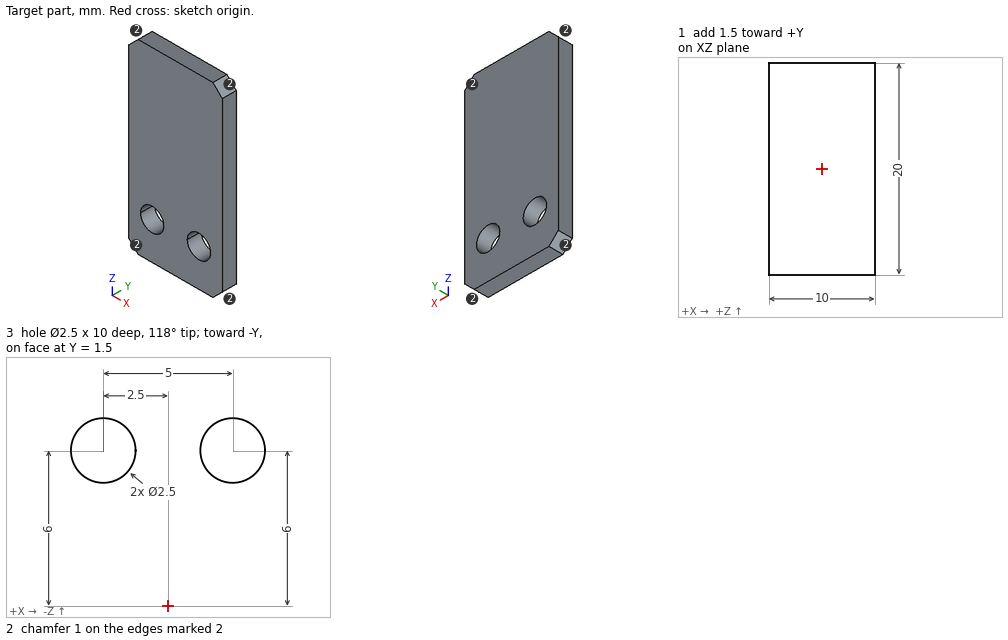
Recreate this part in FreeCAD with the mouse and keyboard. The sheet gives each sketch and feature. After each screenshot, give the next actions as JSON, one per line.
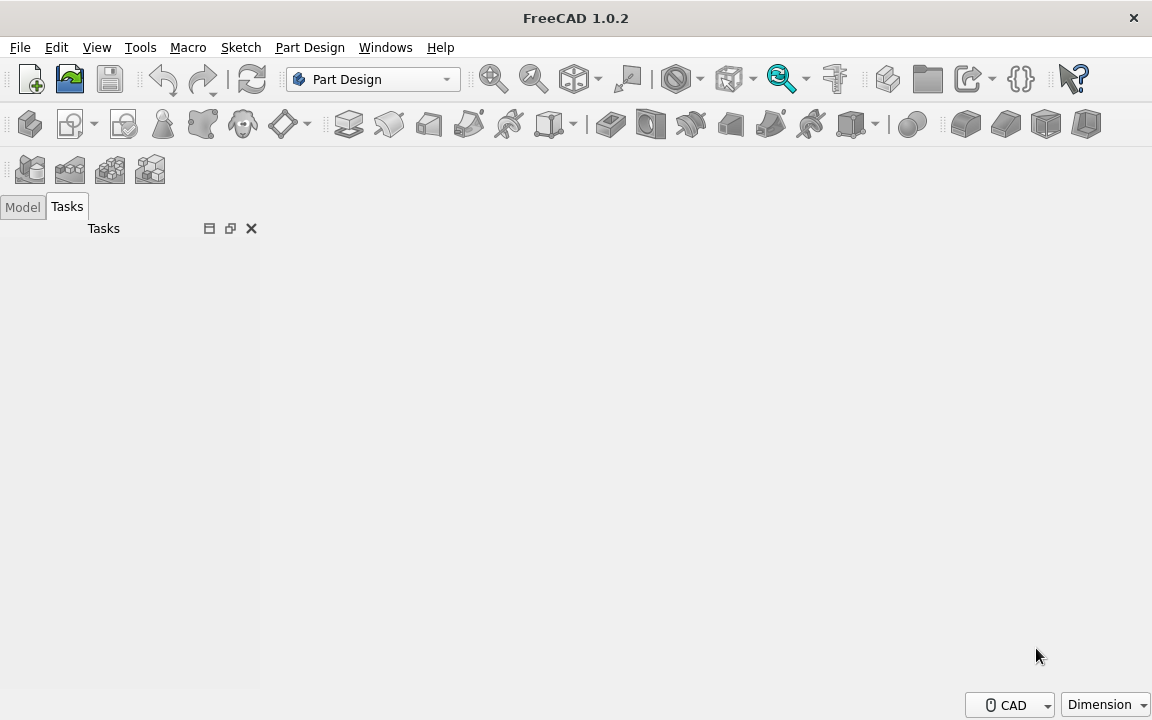
{"action": "left_click", "coordinate": [30, 80]}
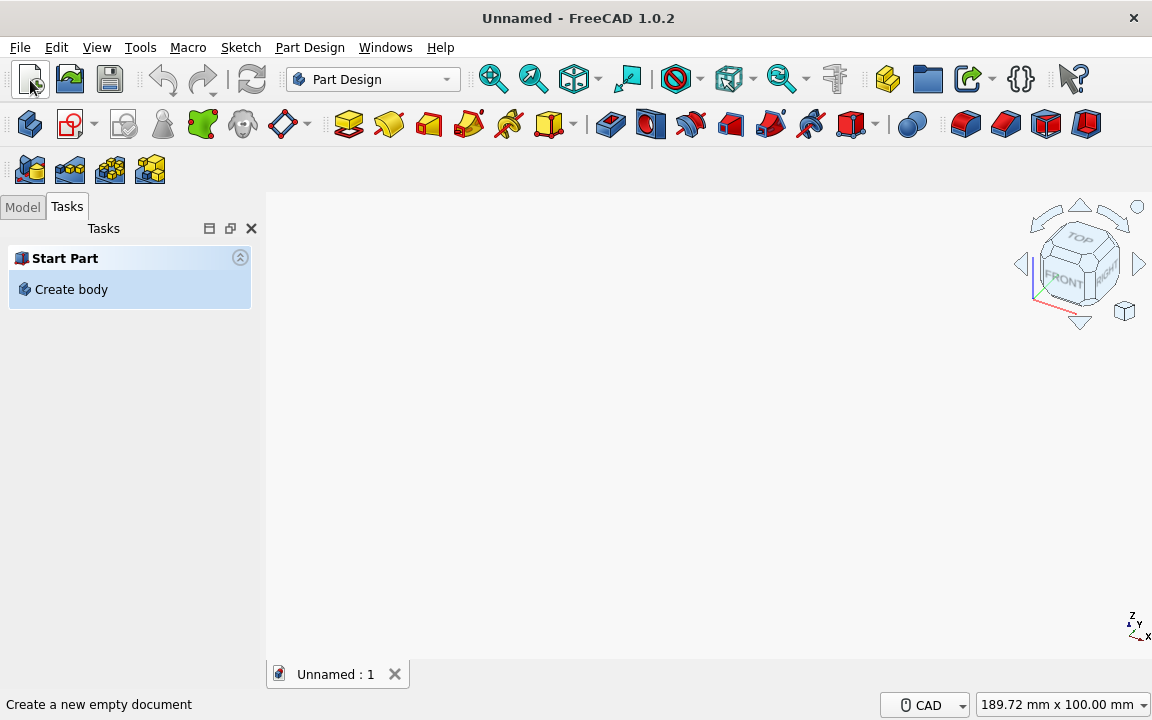
{"action": "left_click", "coordinate": [70, 124]}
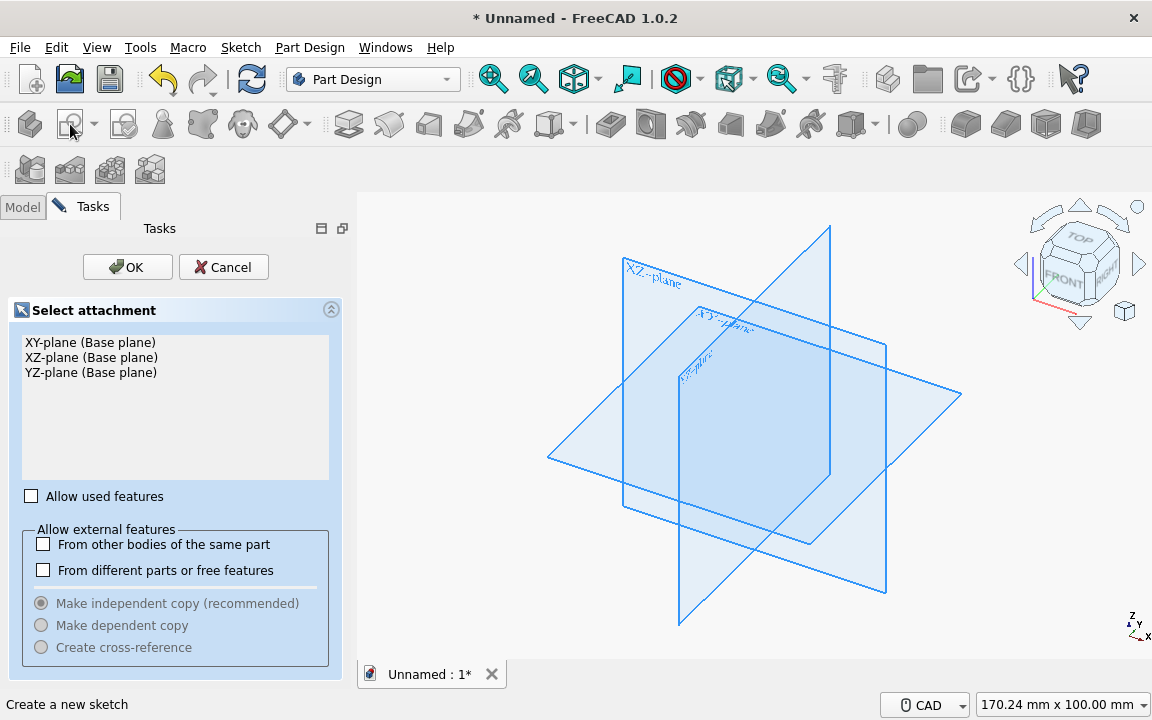
{"action": "left_click", "coordinate": [82, 358]}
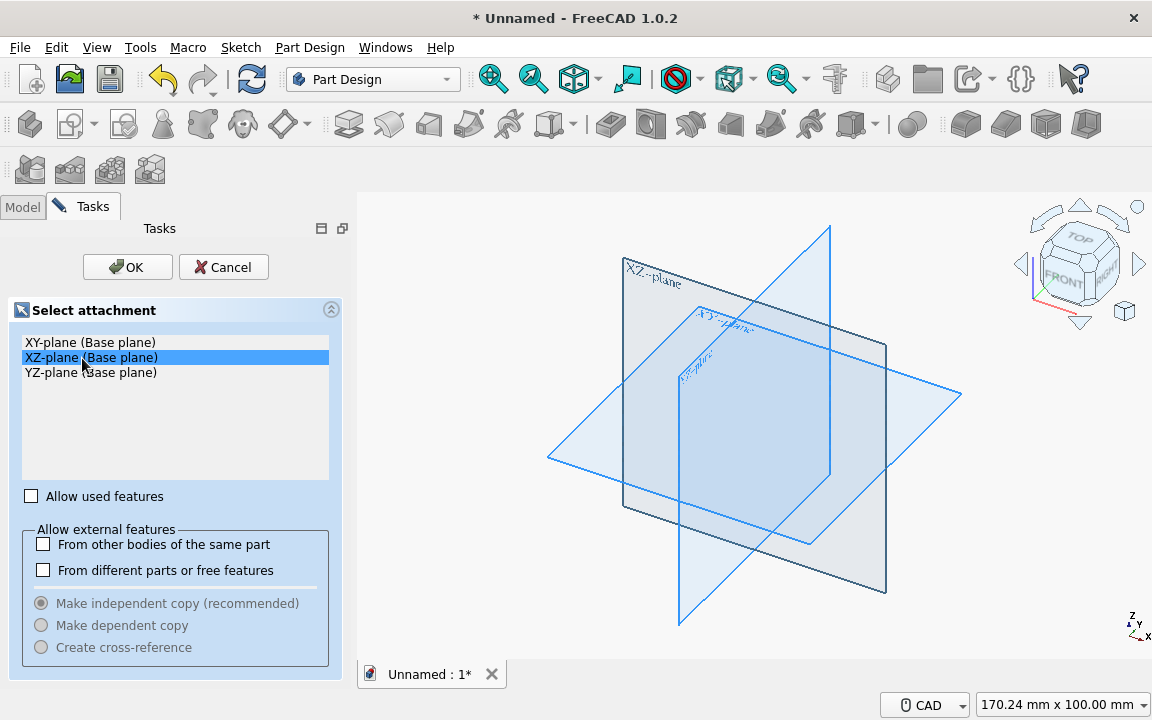
{"action": "left_click", "coordinate": [128, 267]}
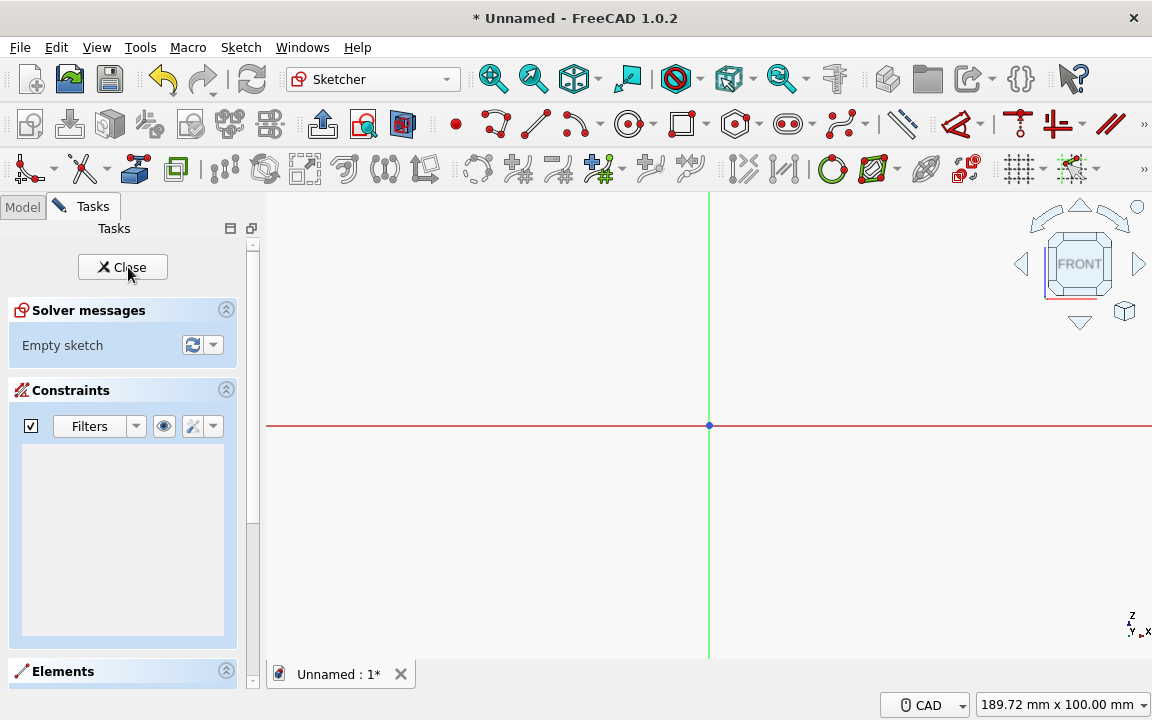
{"action": "scroll", "coordinate": [739, 426], "scroll_direction": "up", "scroll_amount": 6}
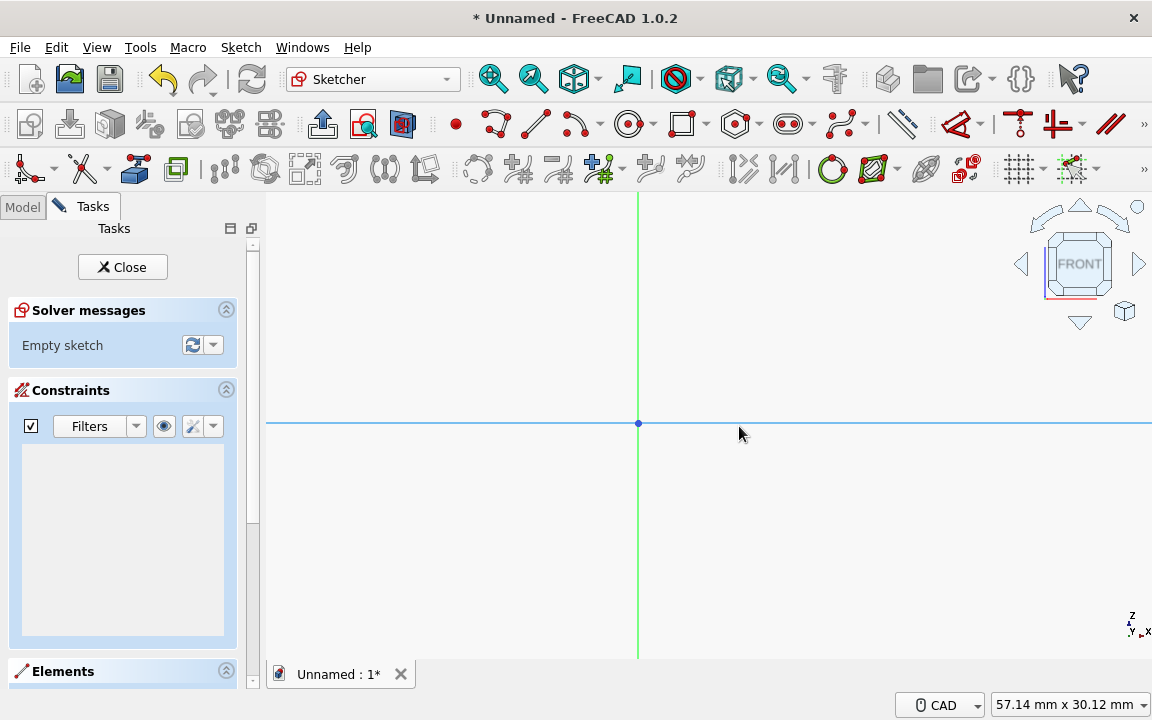
{"action": "left_click", "coordinate": [708, 124]}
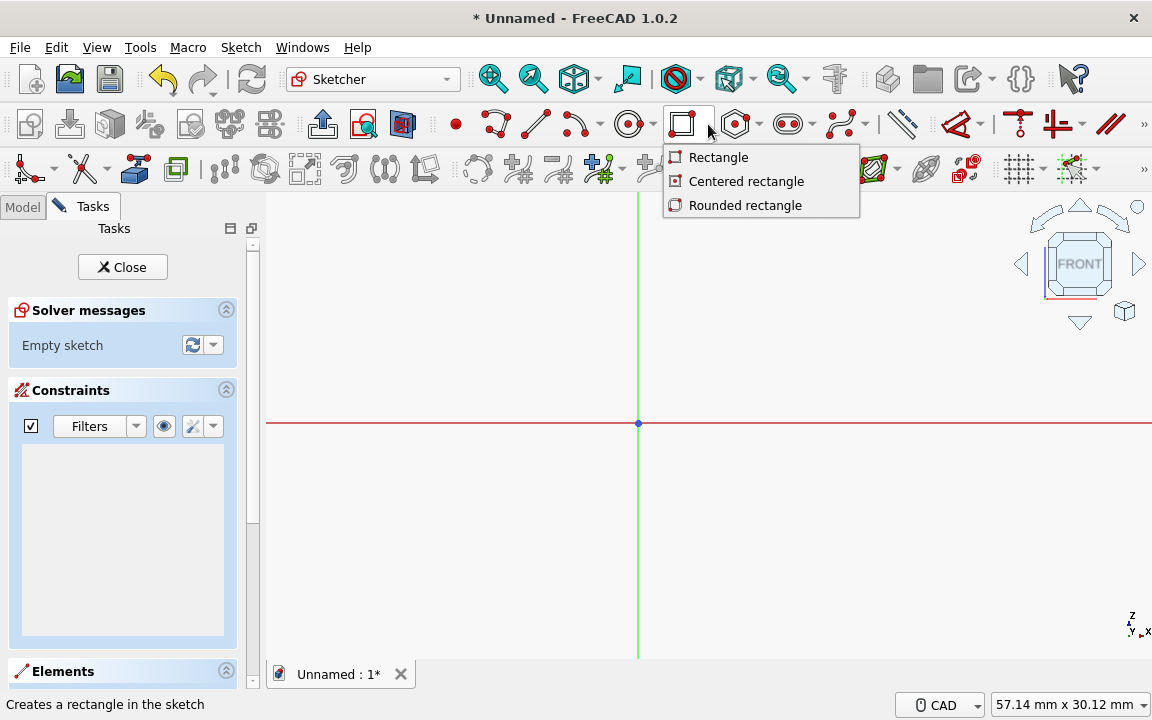
{"action": "left_click", "coordinate": [762, 181]}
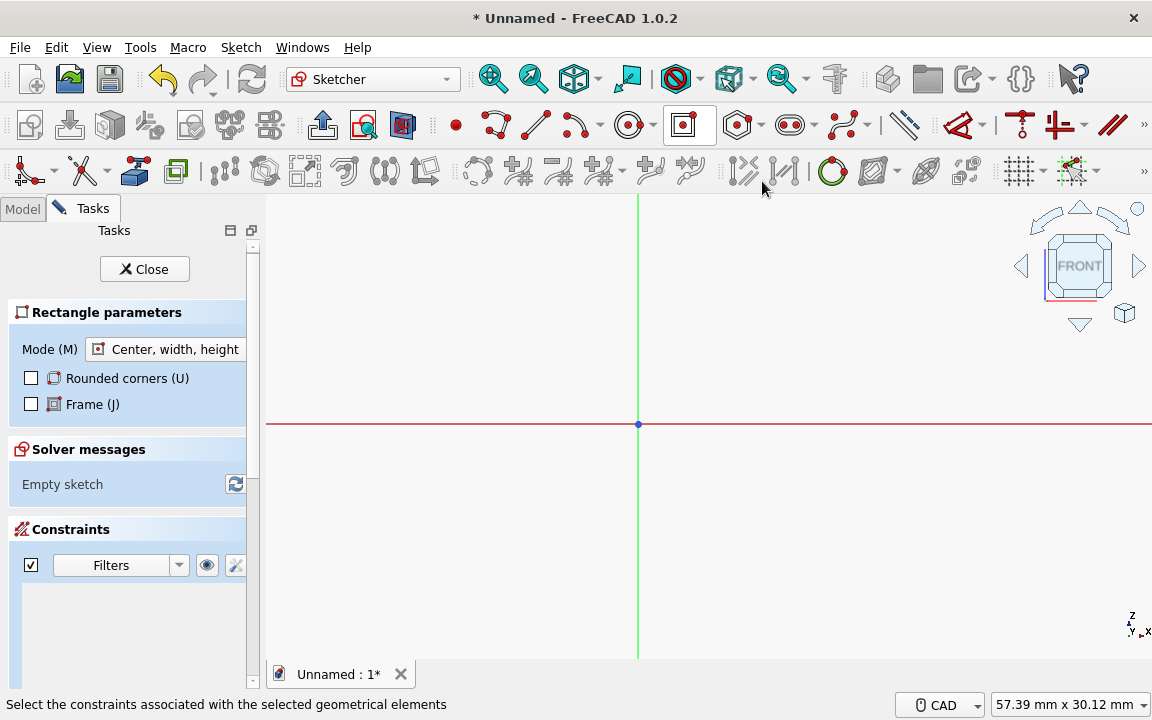
{"action": "left_click", "coordinate": [638, 424]}
{"action": "left_click", "coordinate": [716, 270]}
{"action": "key", "text": "Escape"}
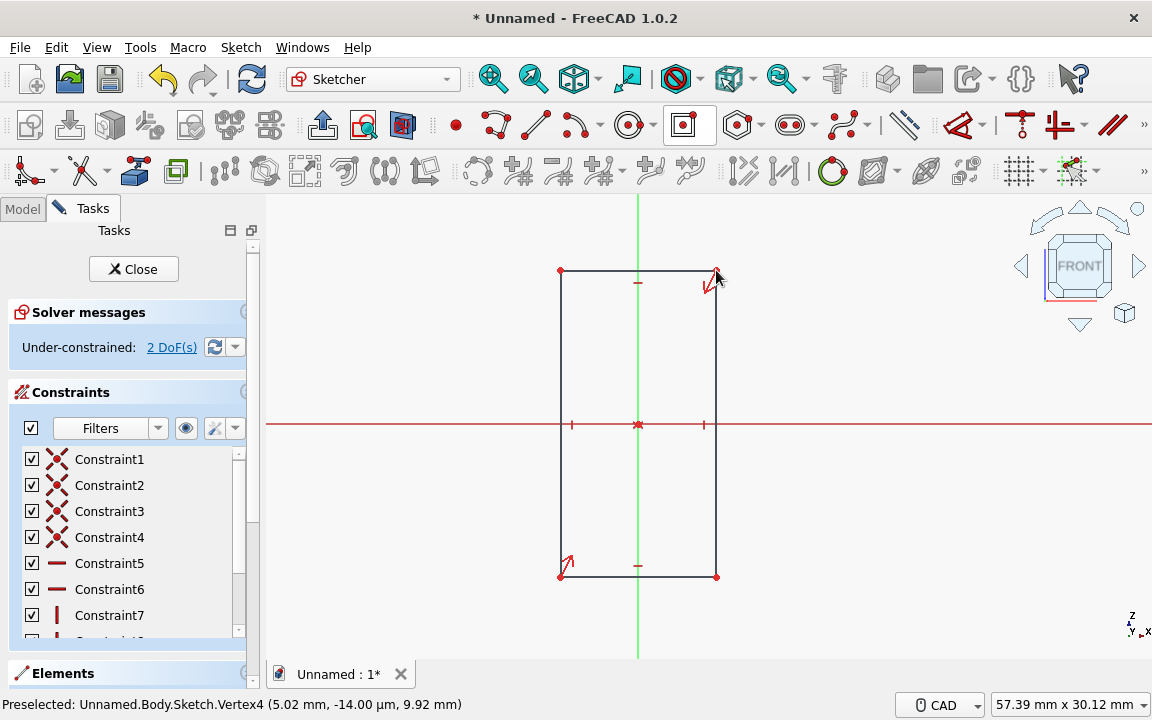
{"action": "left_click", "coordinate": [958, 126]}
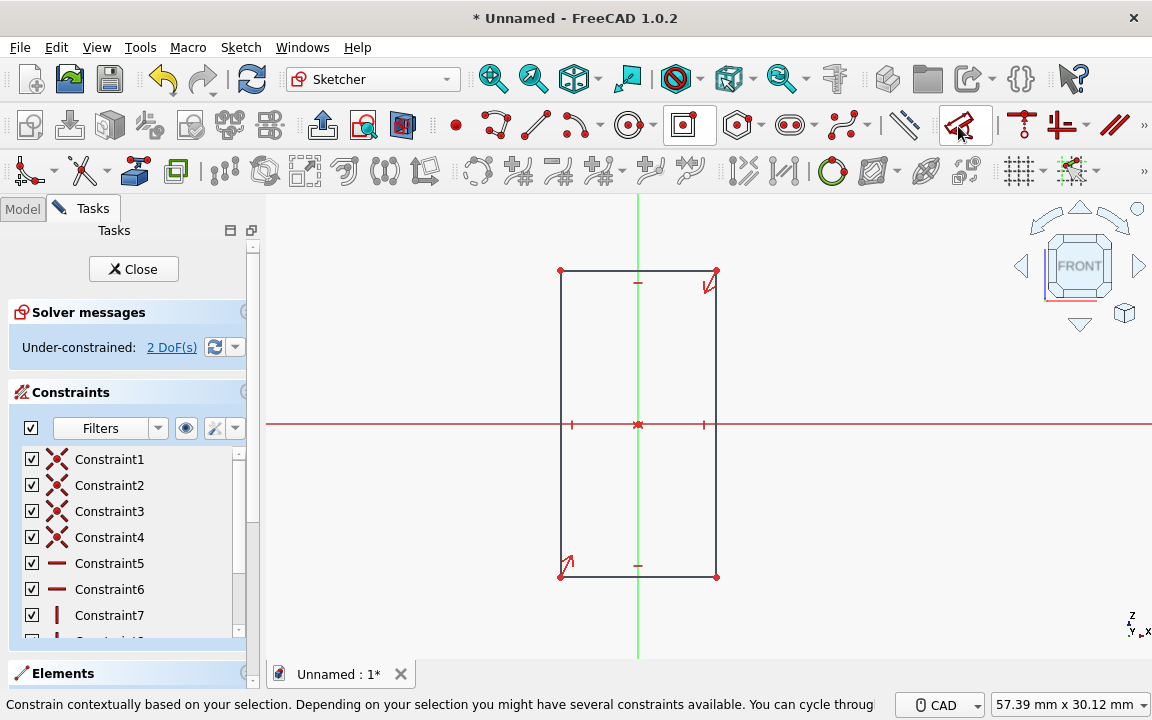
{"action": "left_click", "coordinate": [607, 577]}
{"action": "left_click", "coordinate": [603, 611]}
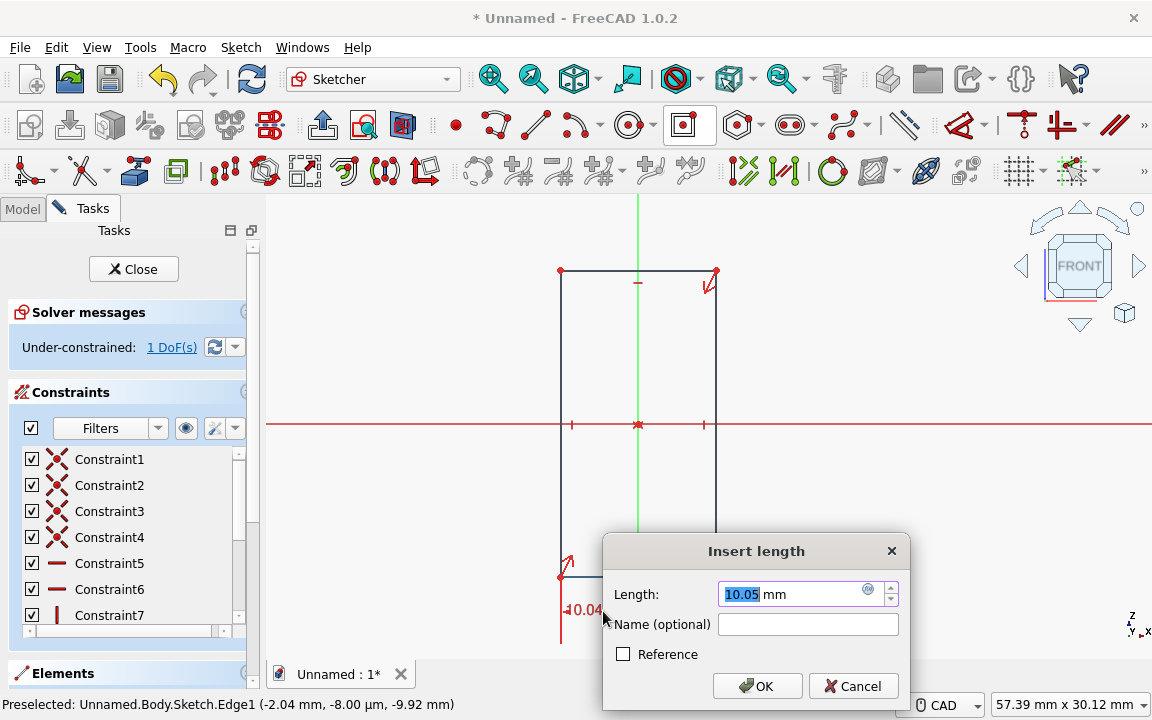
{"action": "type", "text": "10"}
{"action": "key", "text": "Return"}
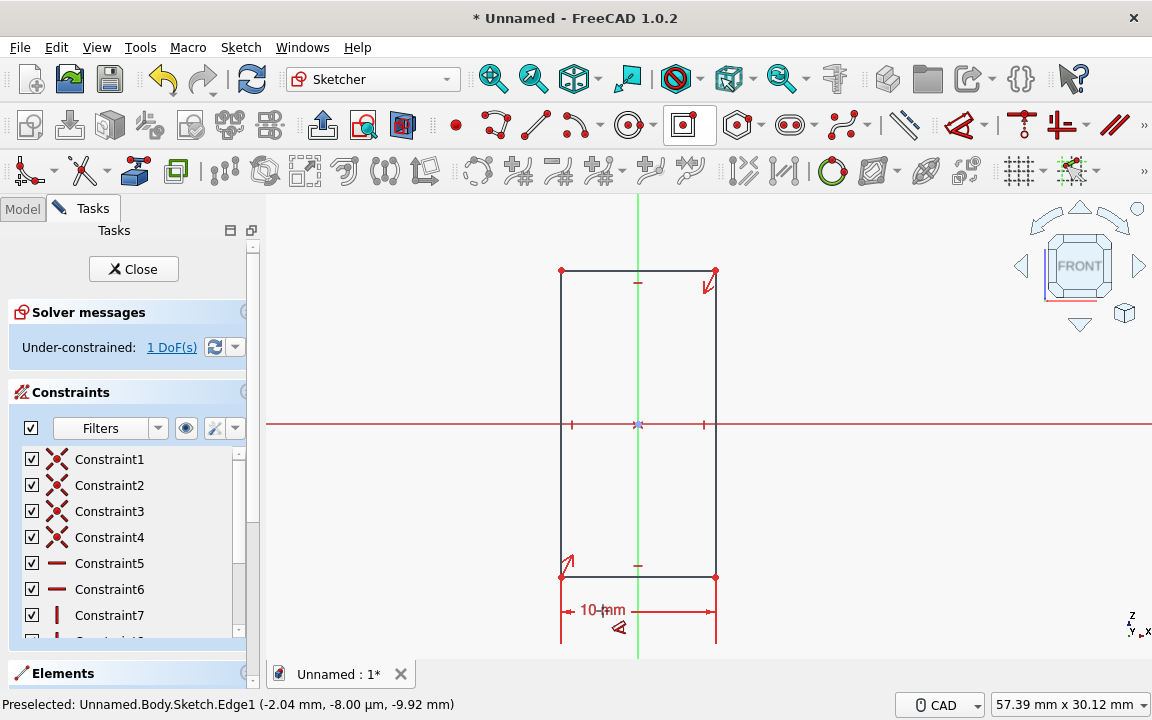
{"action": "left_click", "coordinate": [716, 485]}
{"action": "left_click", "coordinate": [750, 354]}